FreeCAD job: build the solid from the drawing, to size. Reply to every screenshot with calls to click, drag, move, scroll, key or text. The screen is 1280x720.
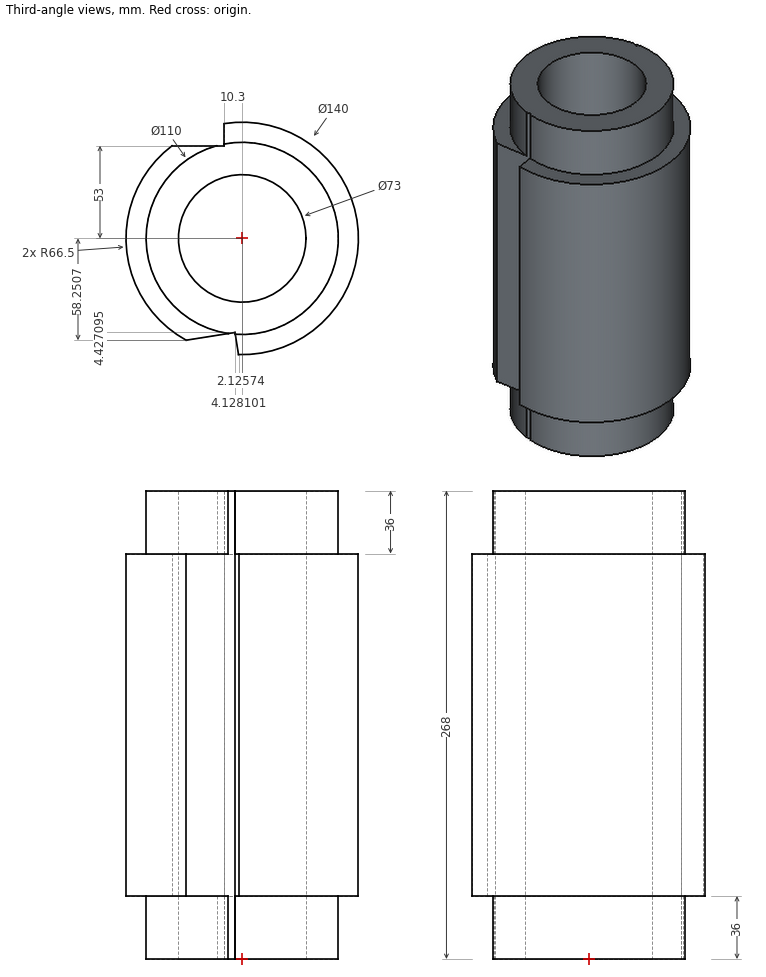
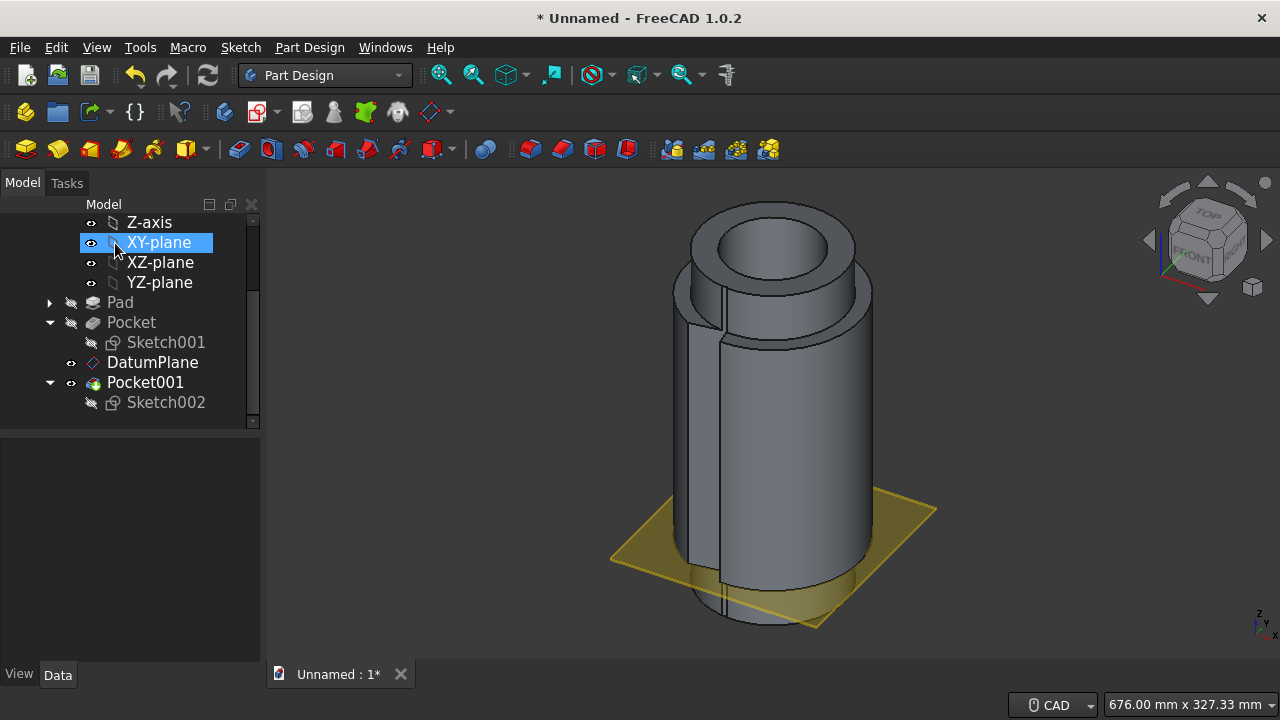
click(116, 363)
key(space)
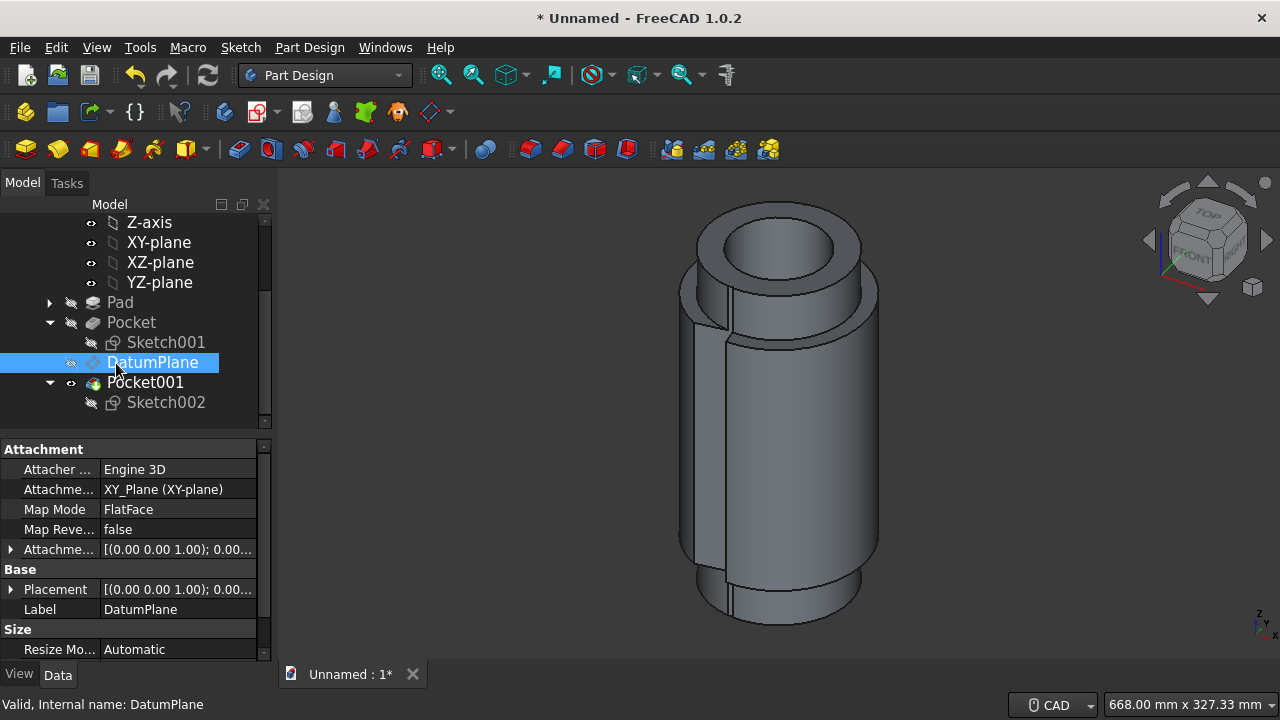
key(0)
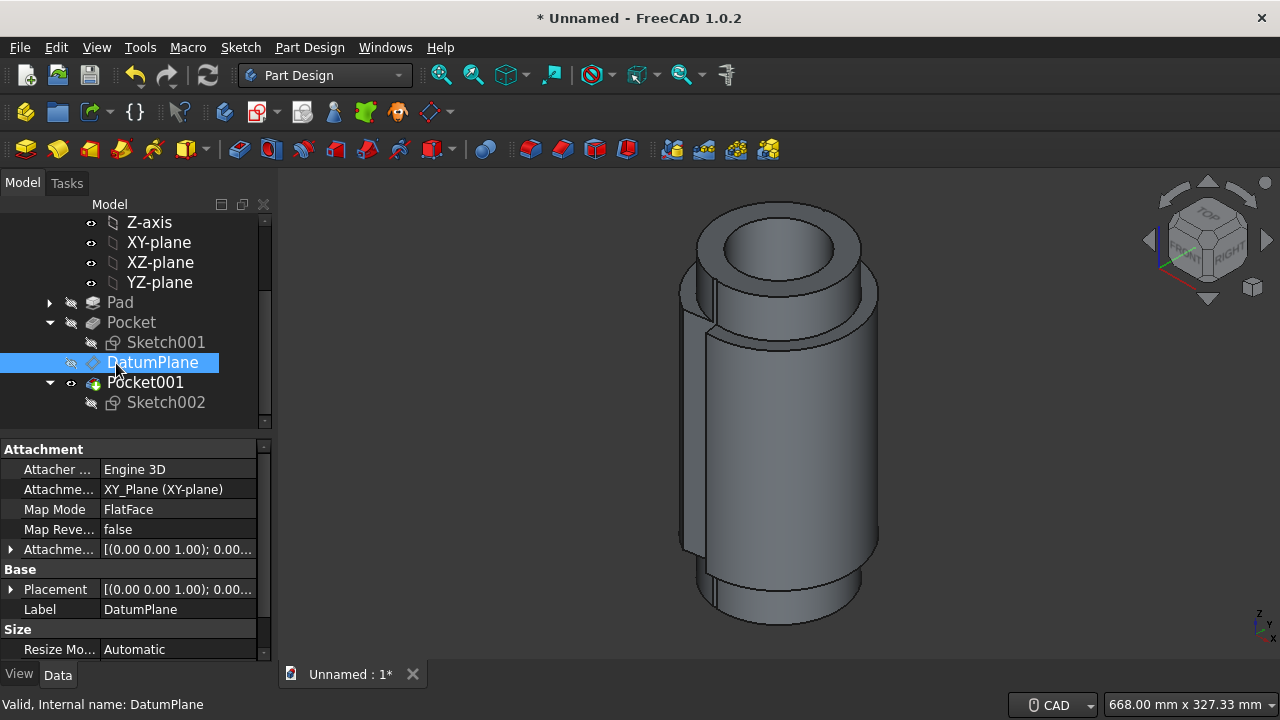
click(442, 76)